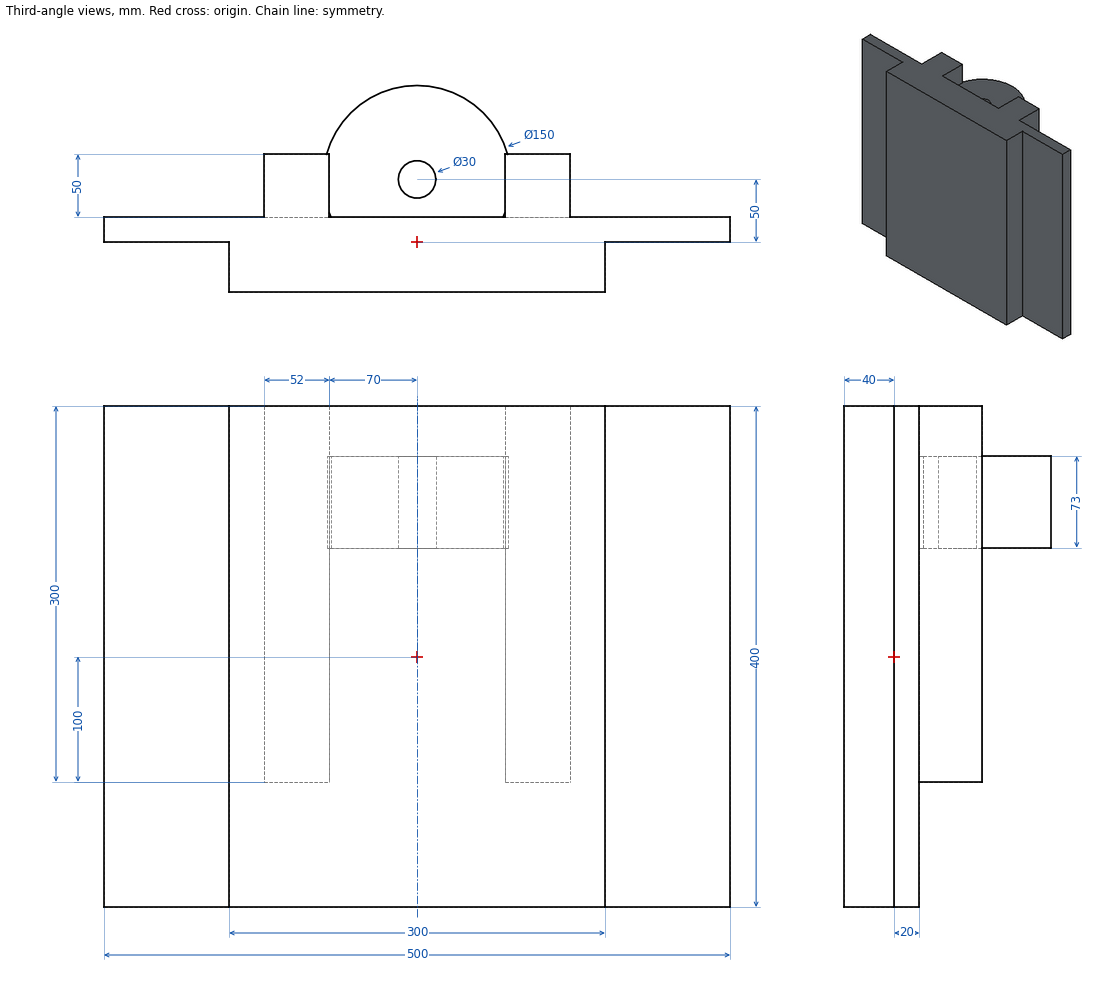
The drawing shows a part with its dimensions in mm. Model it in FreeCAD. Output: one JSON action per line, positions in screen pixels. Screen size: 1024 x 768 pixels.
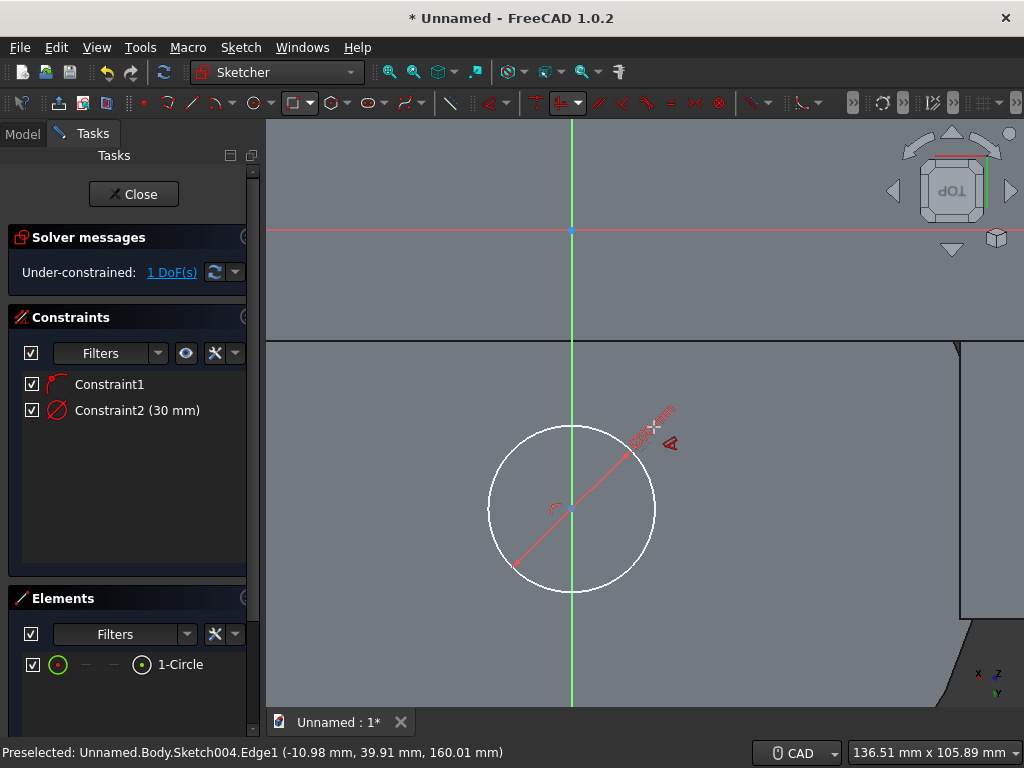
{"action": "left_click", "coordinate": [572, 509]}
{"action": "left_click", "coordinate": [606, 370]}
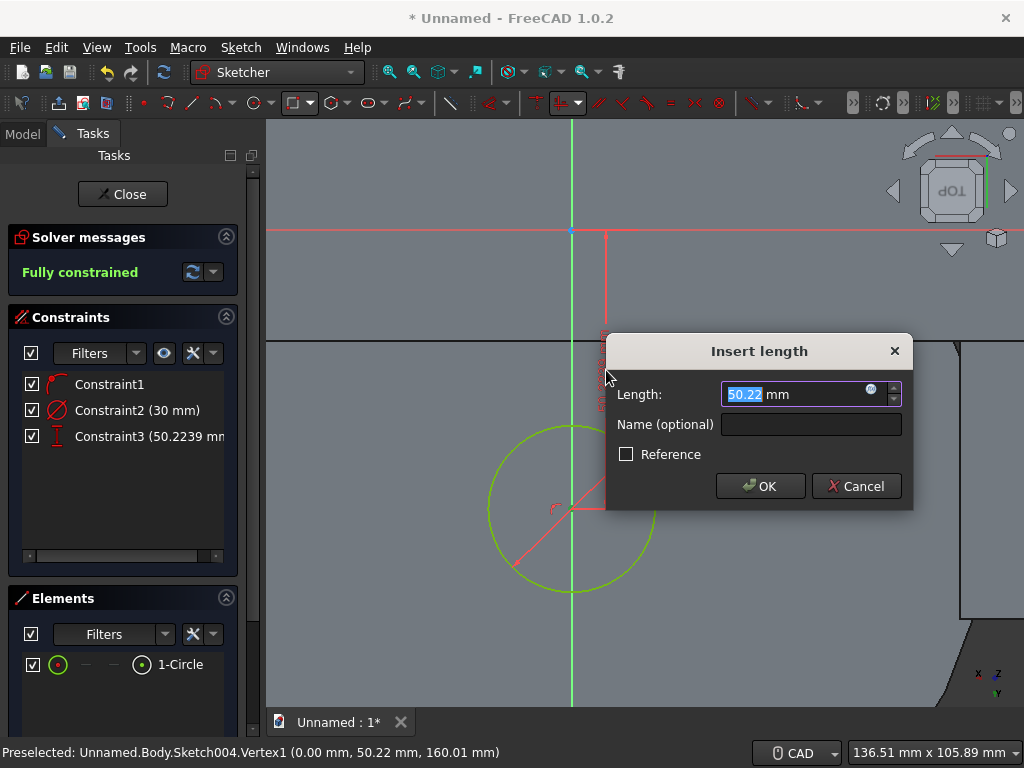
{"action": "type", "text": "50"}
{"action": "key", "text": "Return"}
{"action": "key", "text": "Escape"}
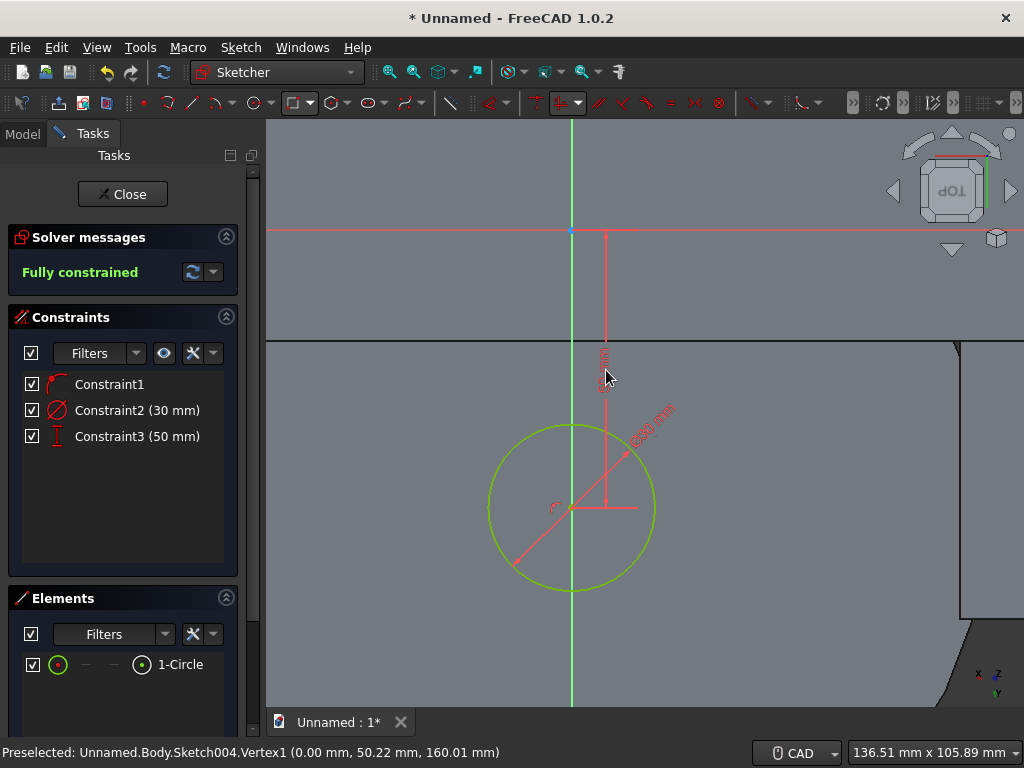
{"action": "left_click", "coordinate": [123, 194]}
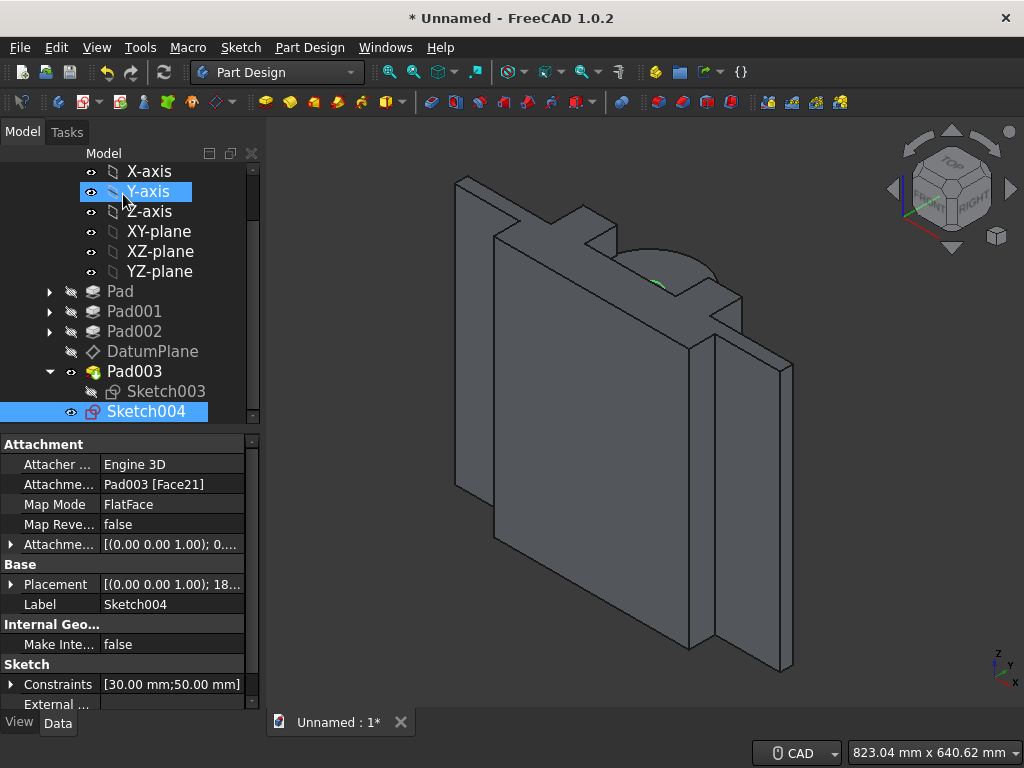
{"action": "left_click", "coordinate": [432, 102]}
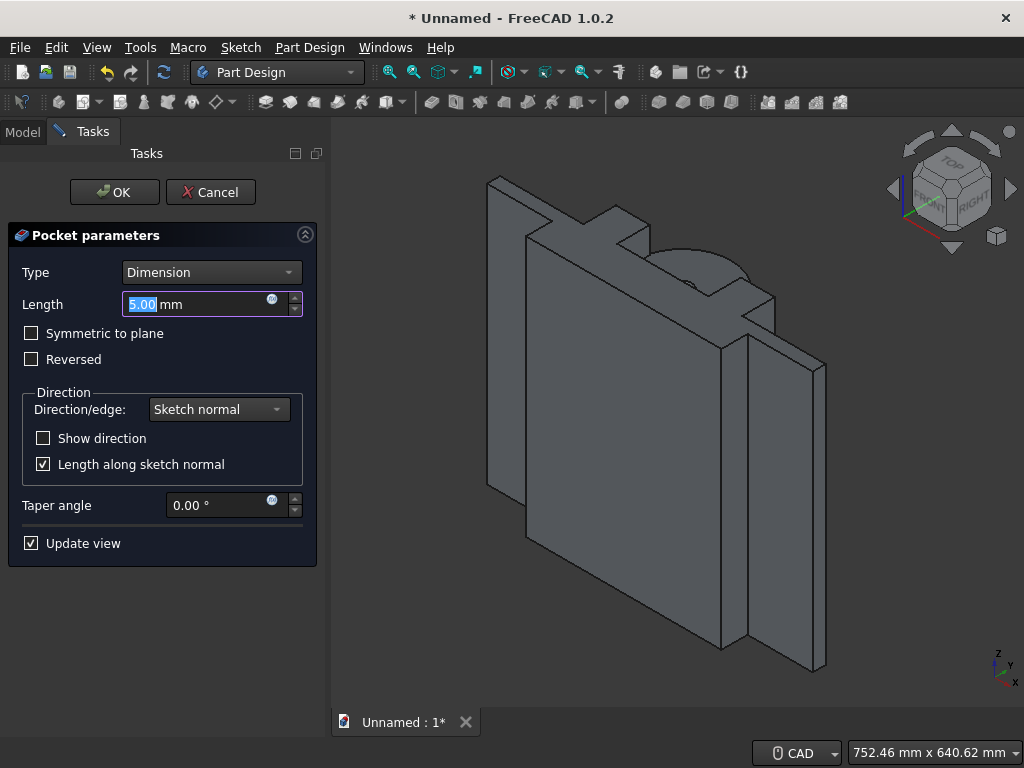
{"action": "left_click", "coordinate": [212, 272]}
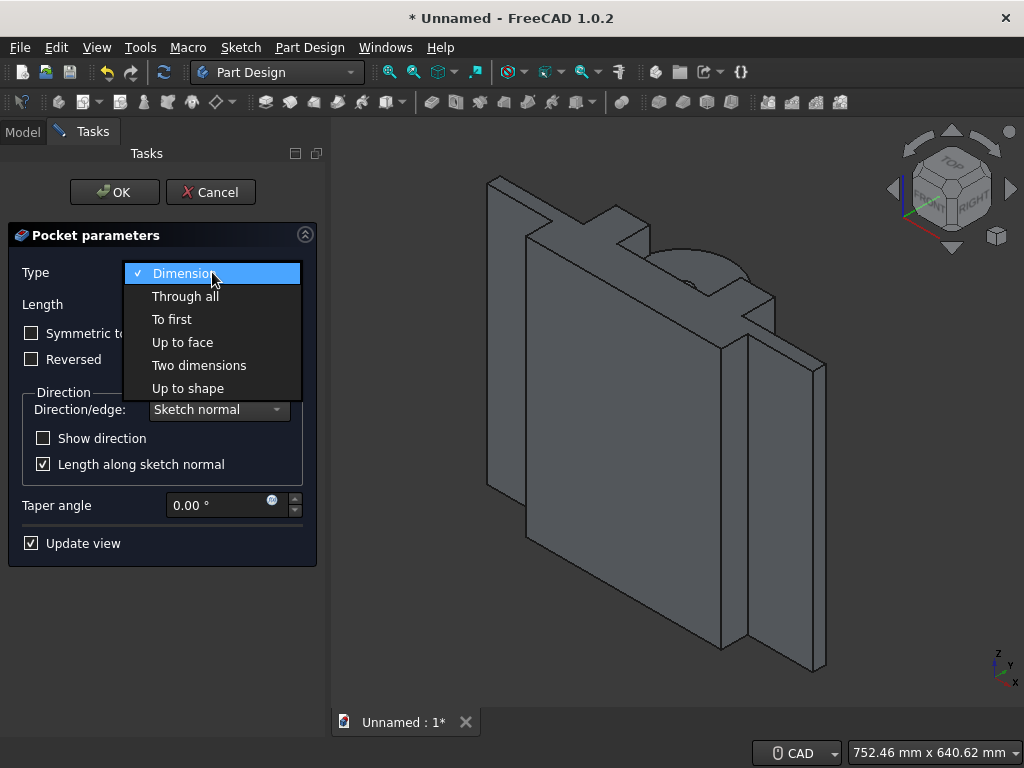
{"action": "left_click", "coordinate": [212, 296]}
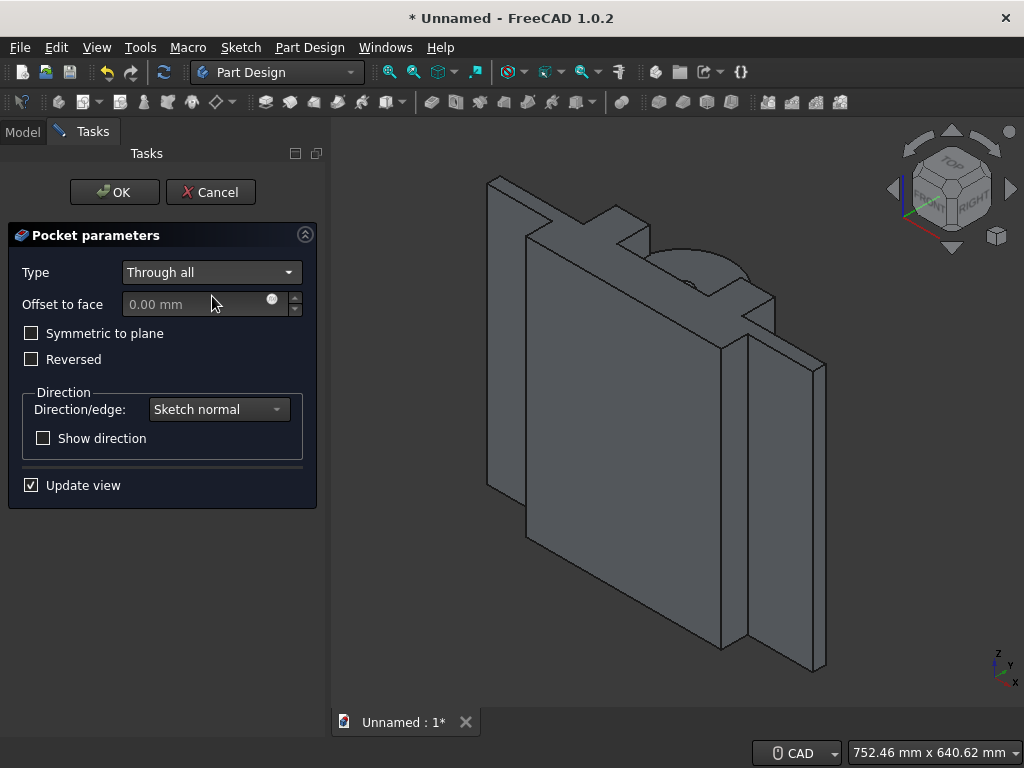
{"action": "left_click", "coordinate": [115, 192]}